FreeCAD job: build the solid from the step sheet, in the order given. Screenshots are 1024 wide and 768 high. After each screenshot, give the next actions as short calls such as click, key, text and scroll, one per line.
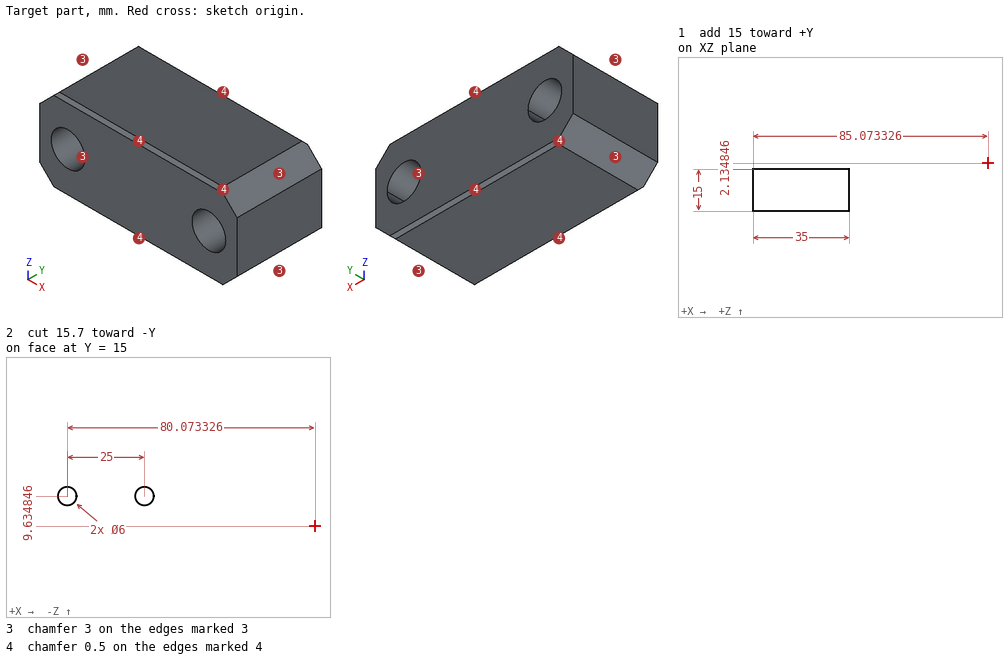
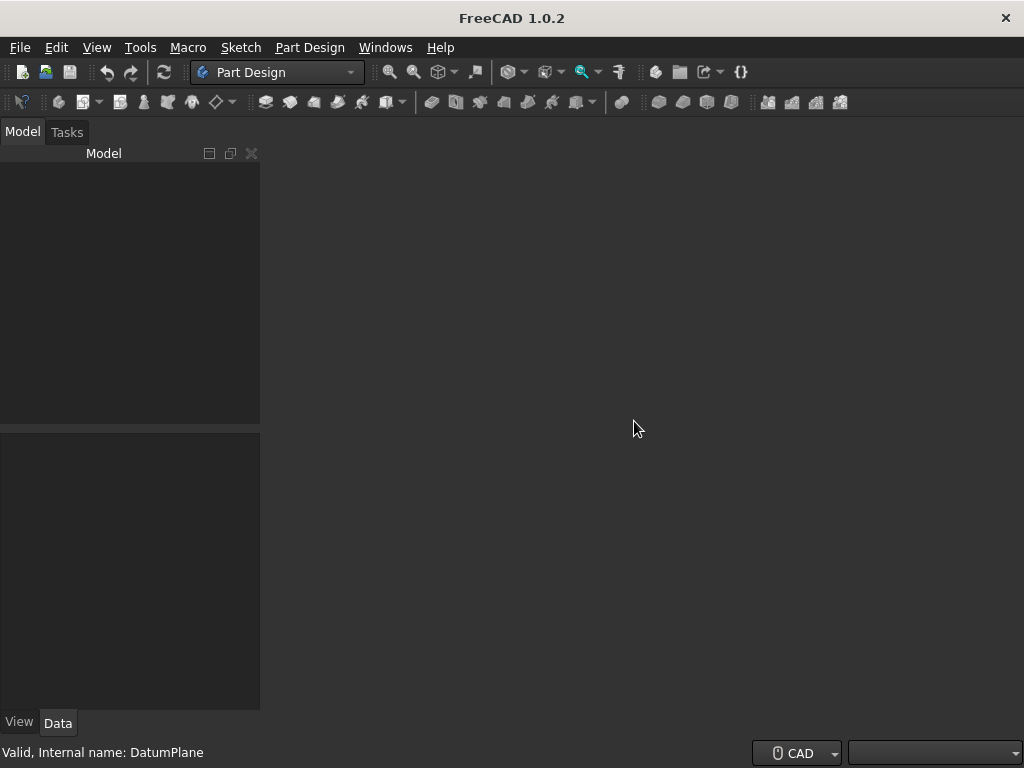
key(ctrl+n)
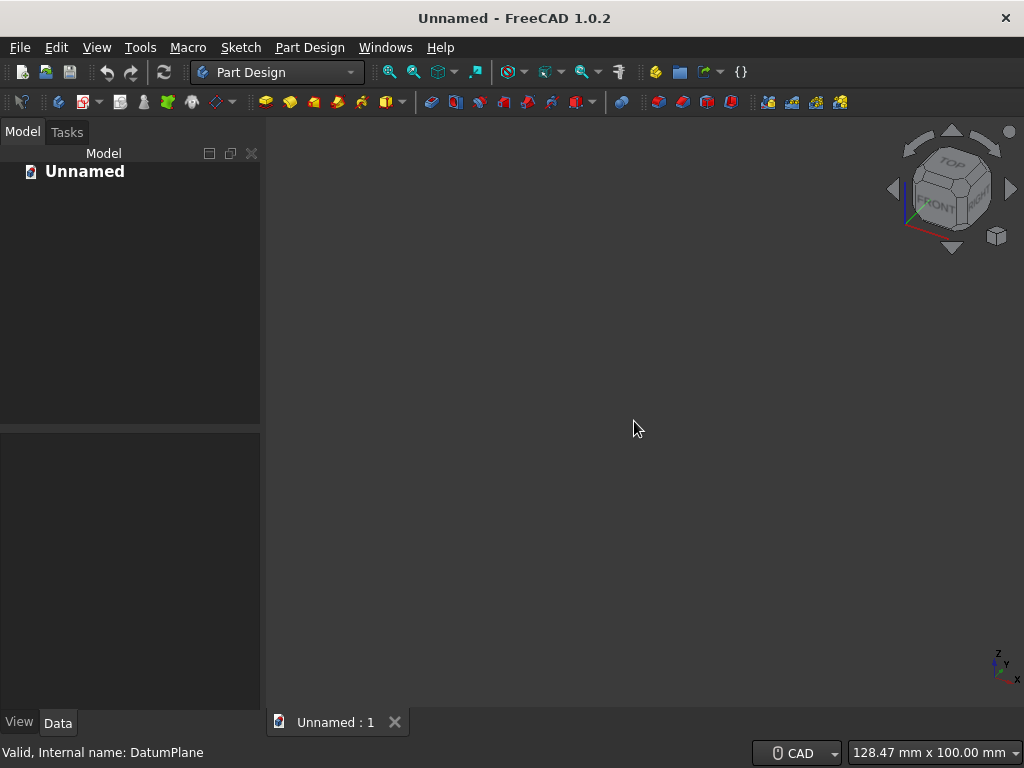
click(84, 102)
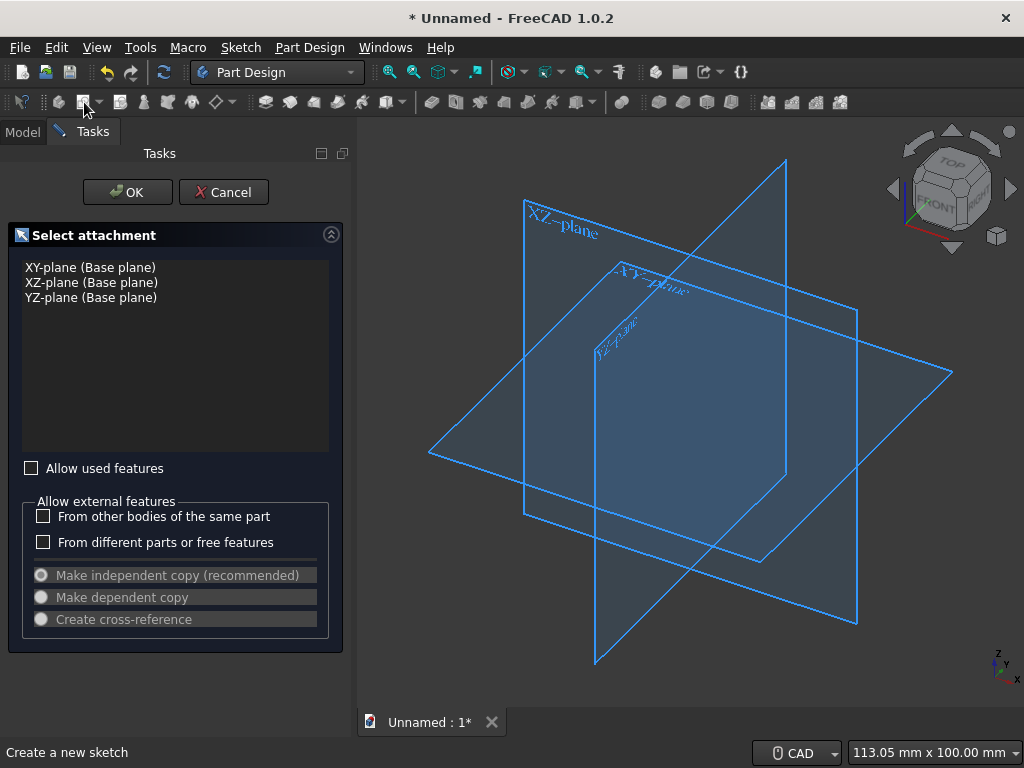
click(82, 282)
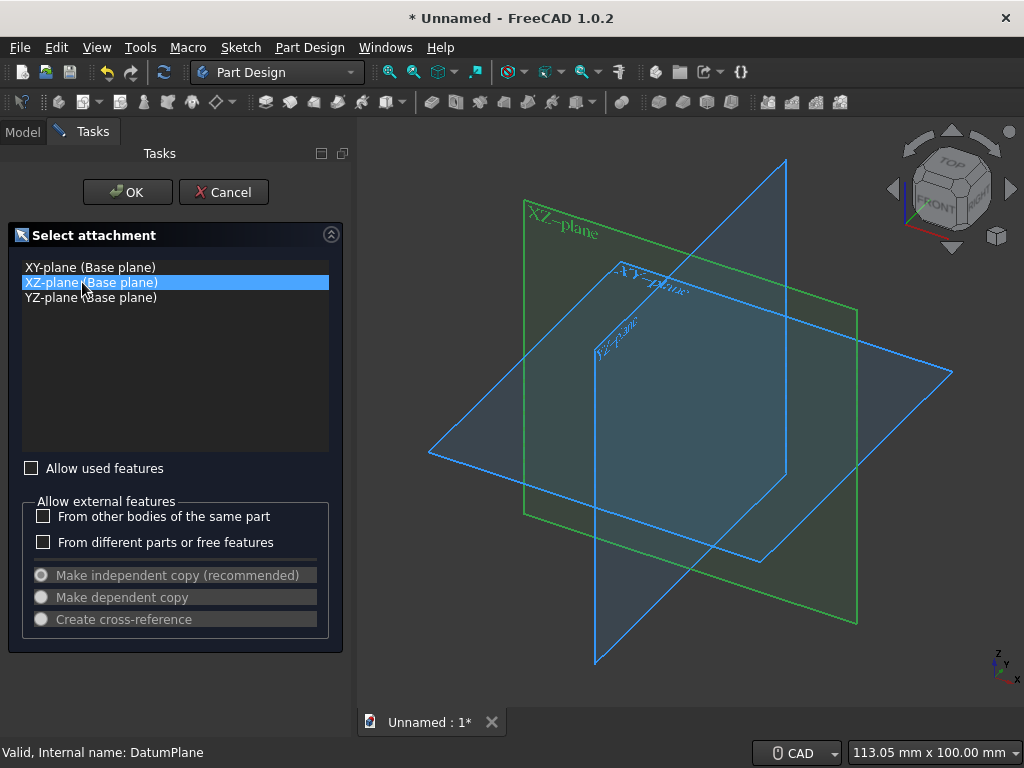
click(128, 192)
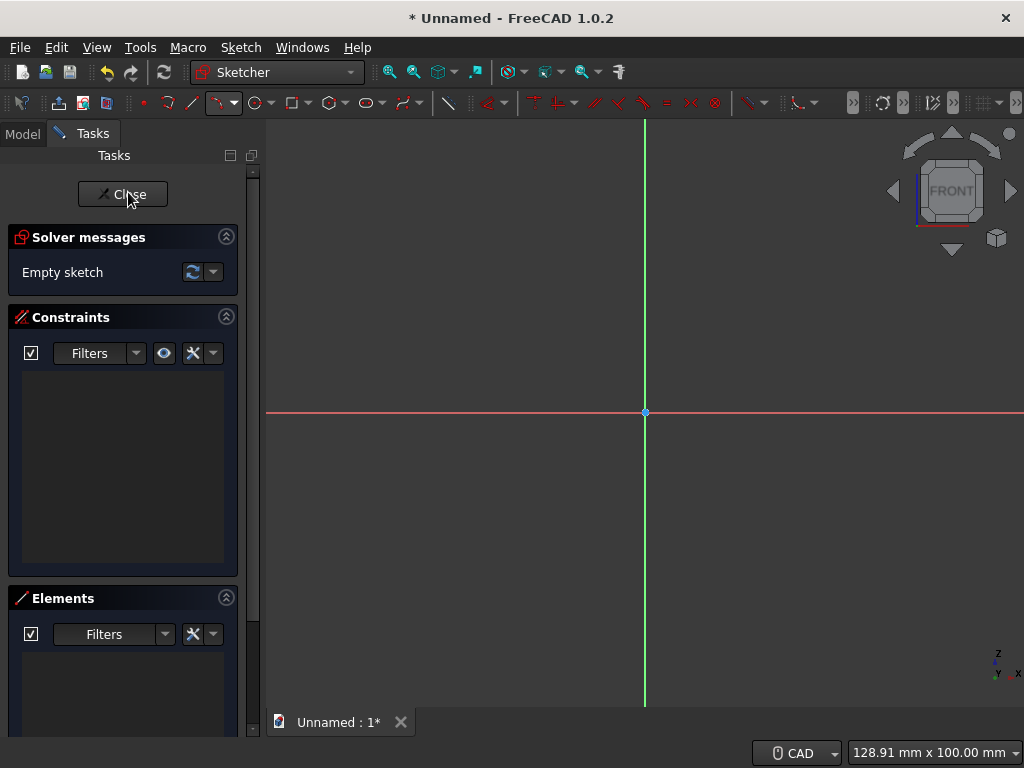
scroll(859, 311, down, 2)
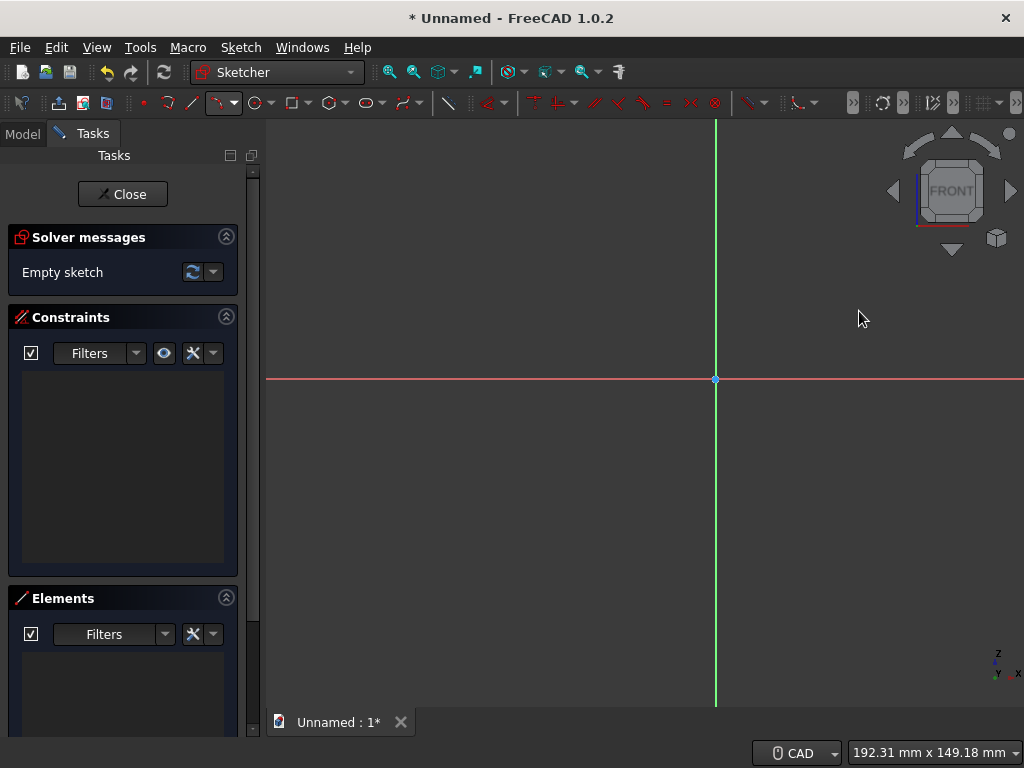
key(g)
key(r)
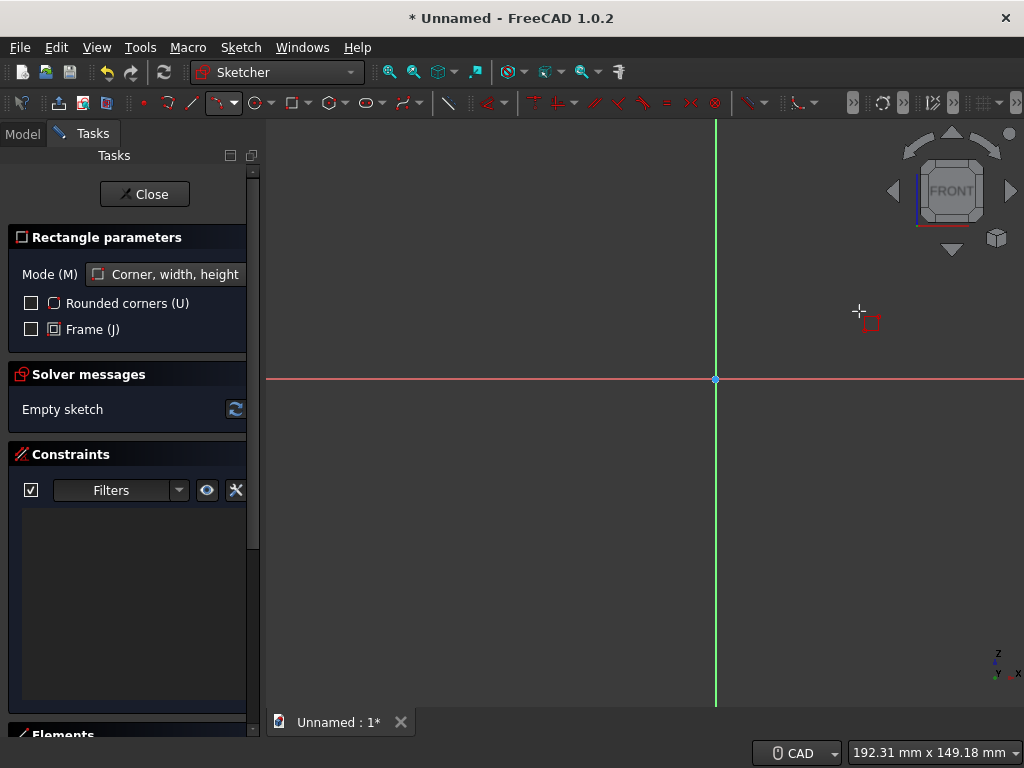
scroll(380, 388, up, 4)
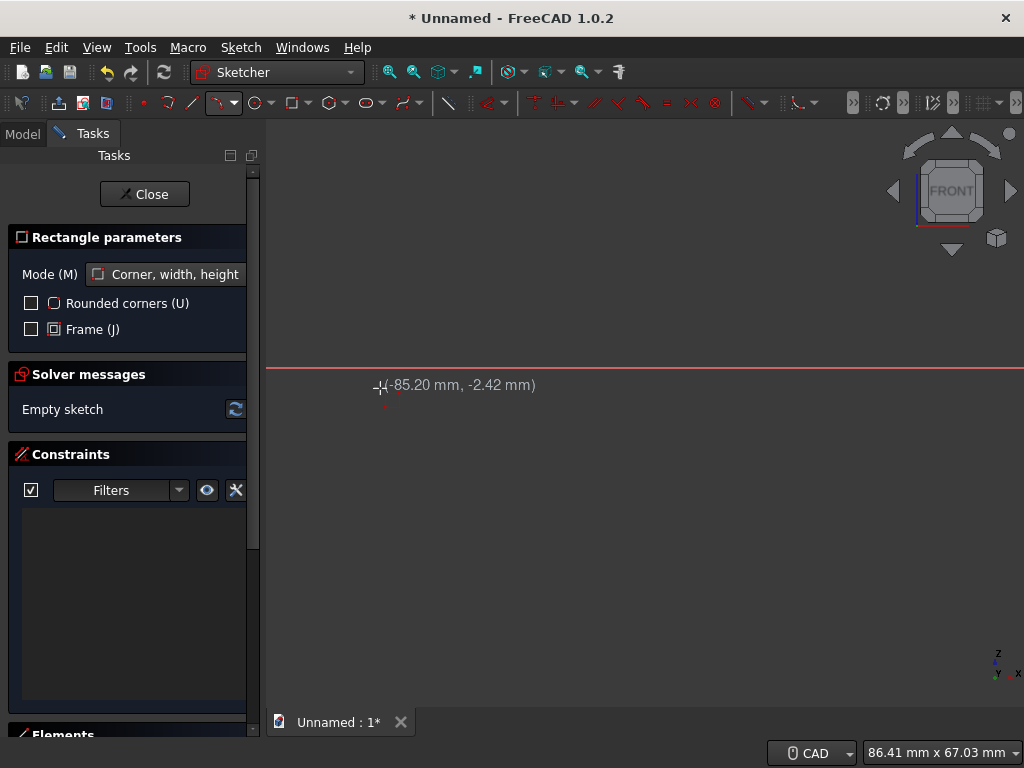
click(381, 387)
click(688, 519)
key(Escape)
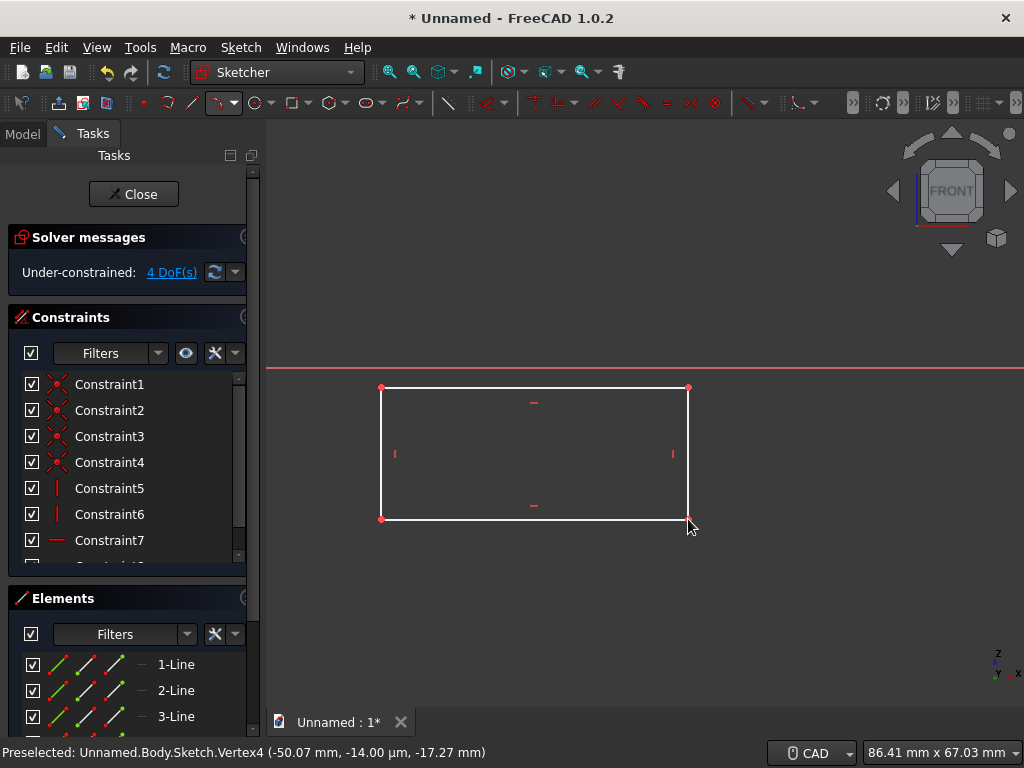
click(381, 428)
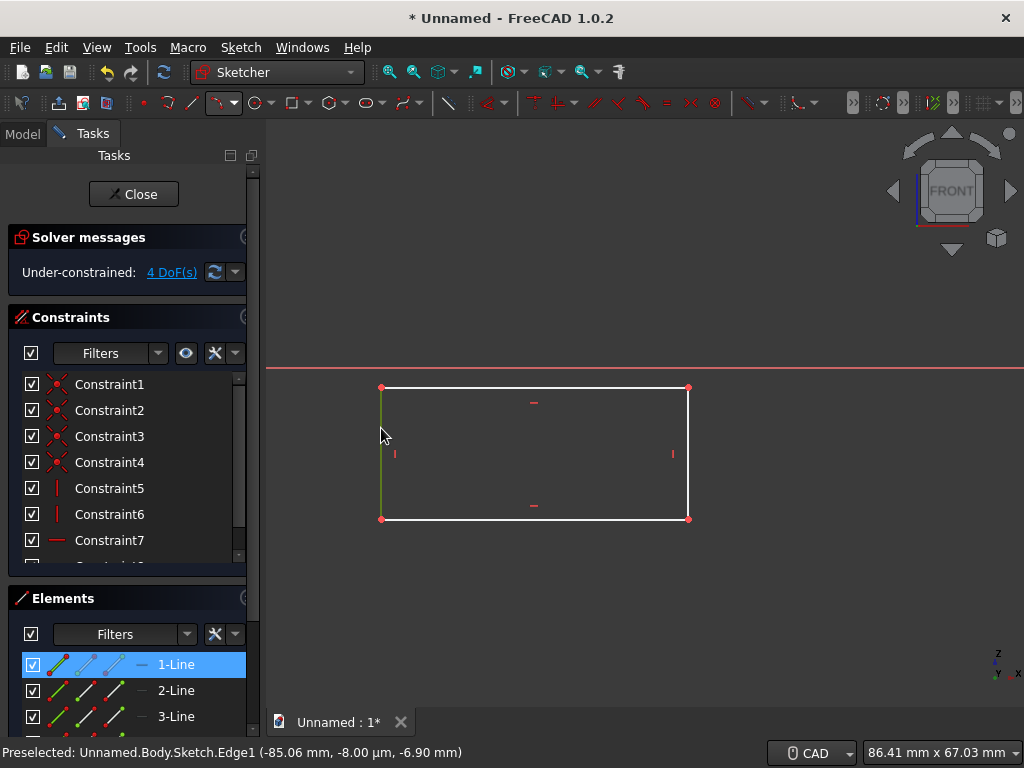
key(i)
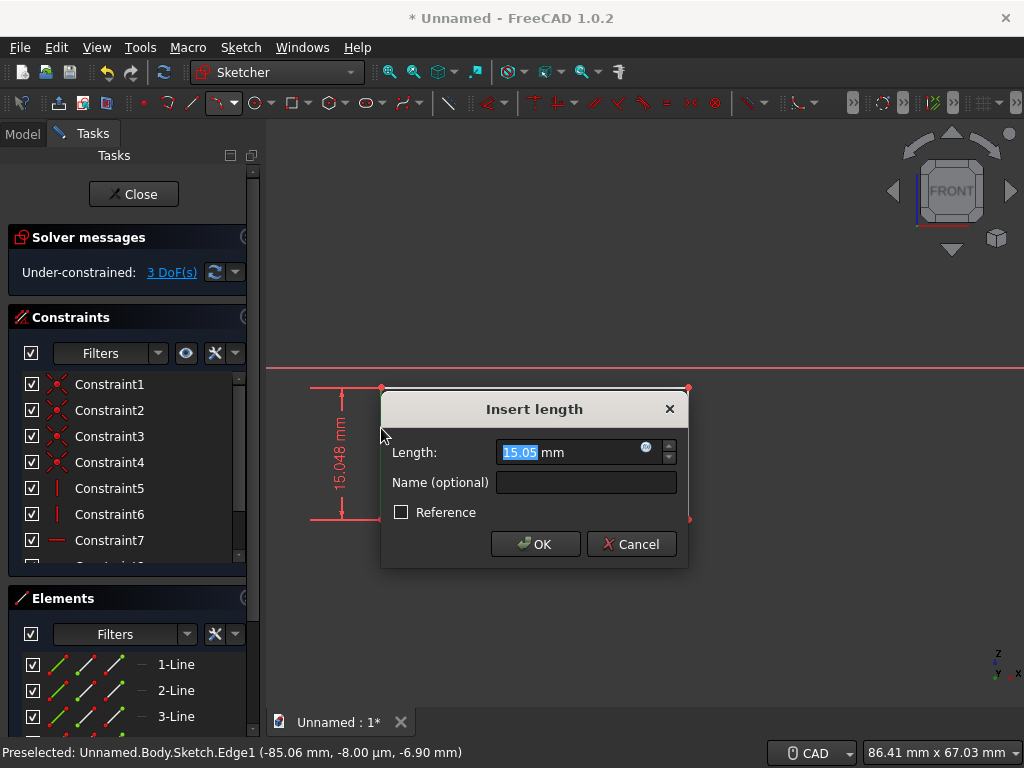
text(15)
key(Return)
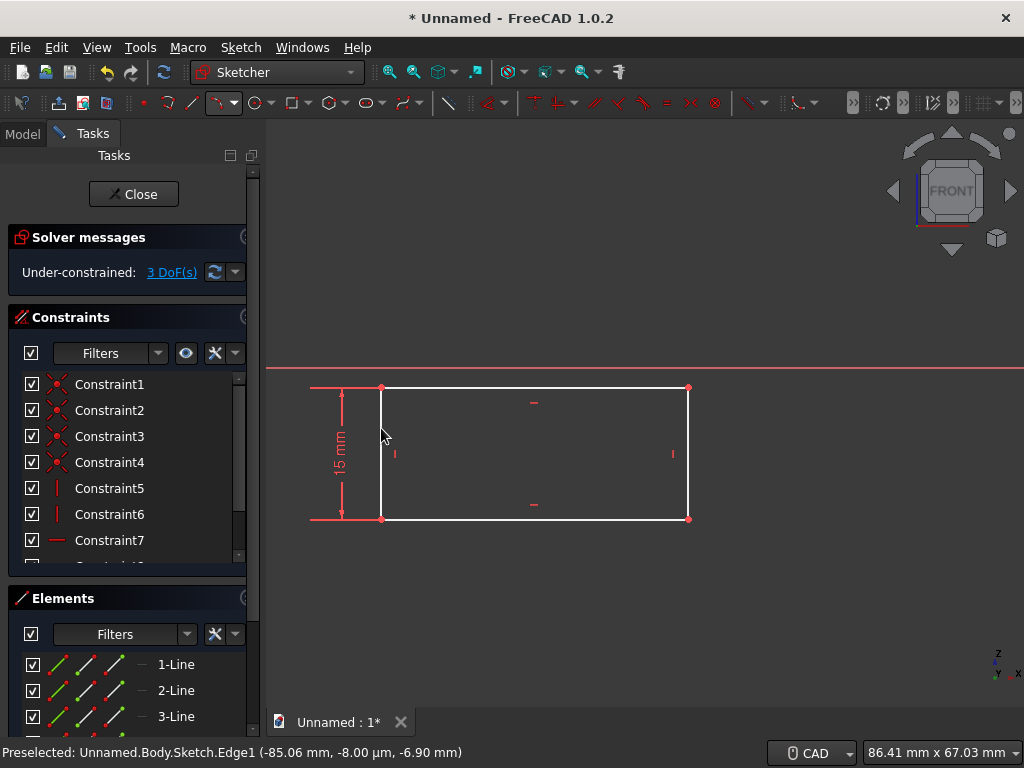
click(473, 520)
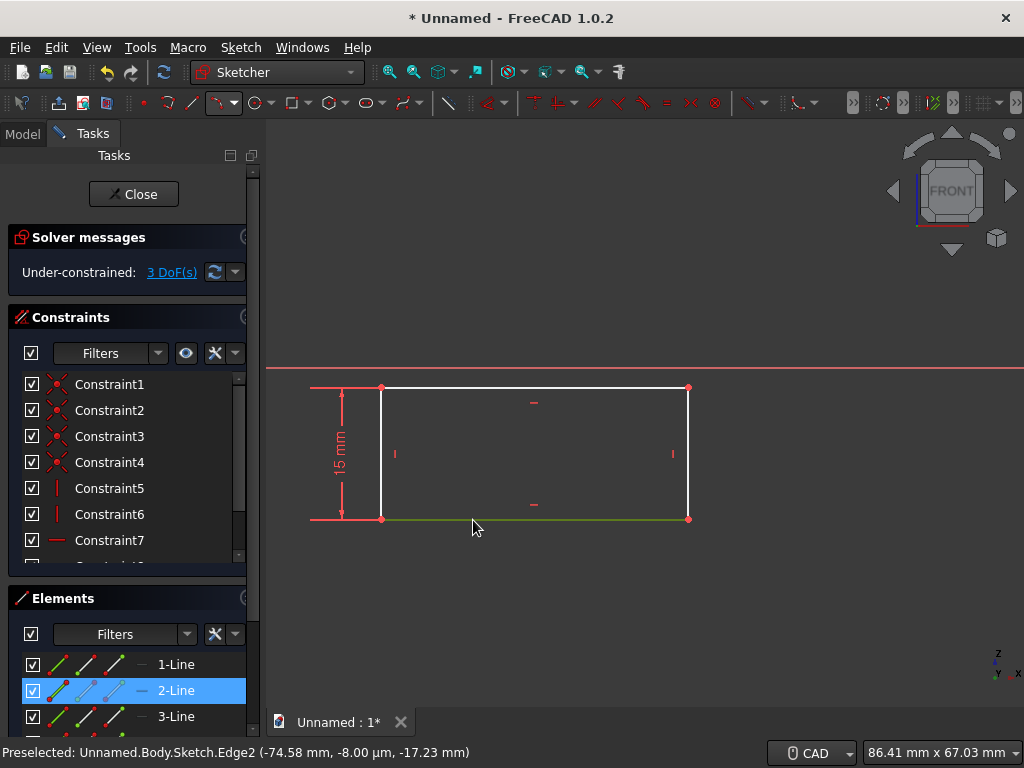
key(l)